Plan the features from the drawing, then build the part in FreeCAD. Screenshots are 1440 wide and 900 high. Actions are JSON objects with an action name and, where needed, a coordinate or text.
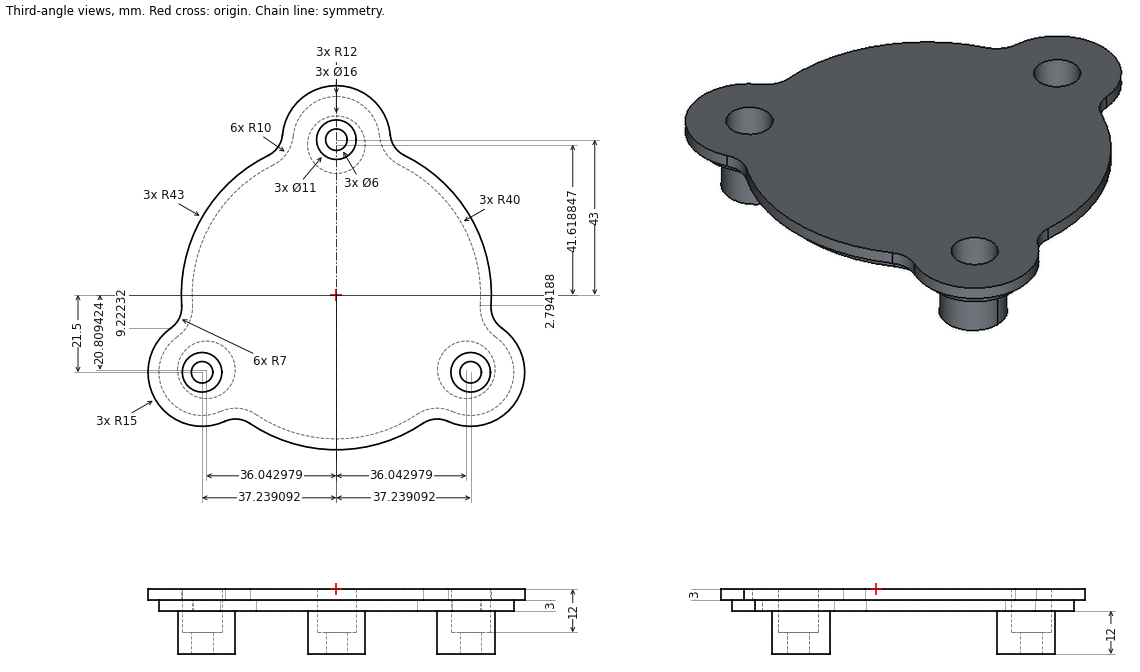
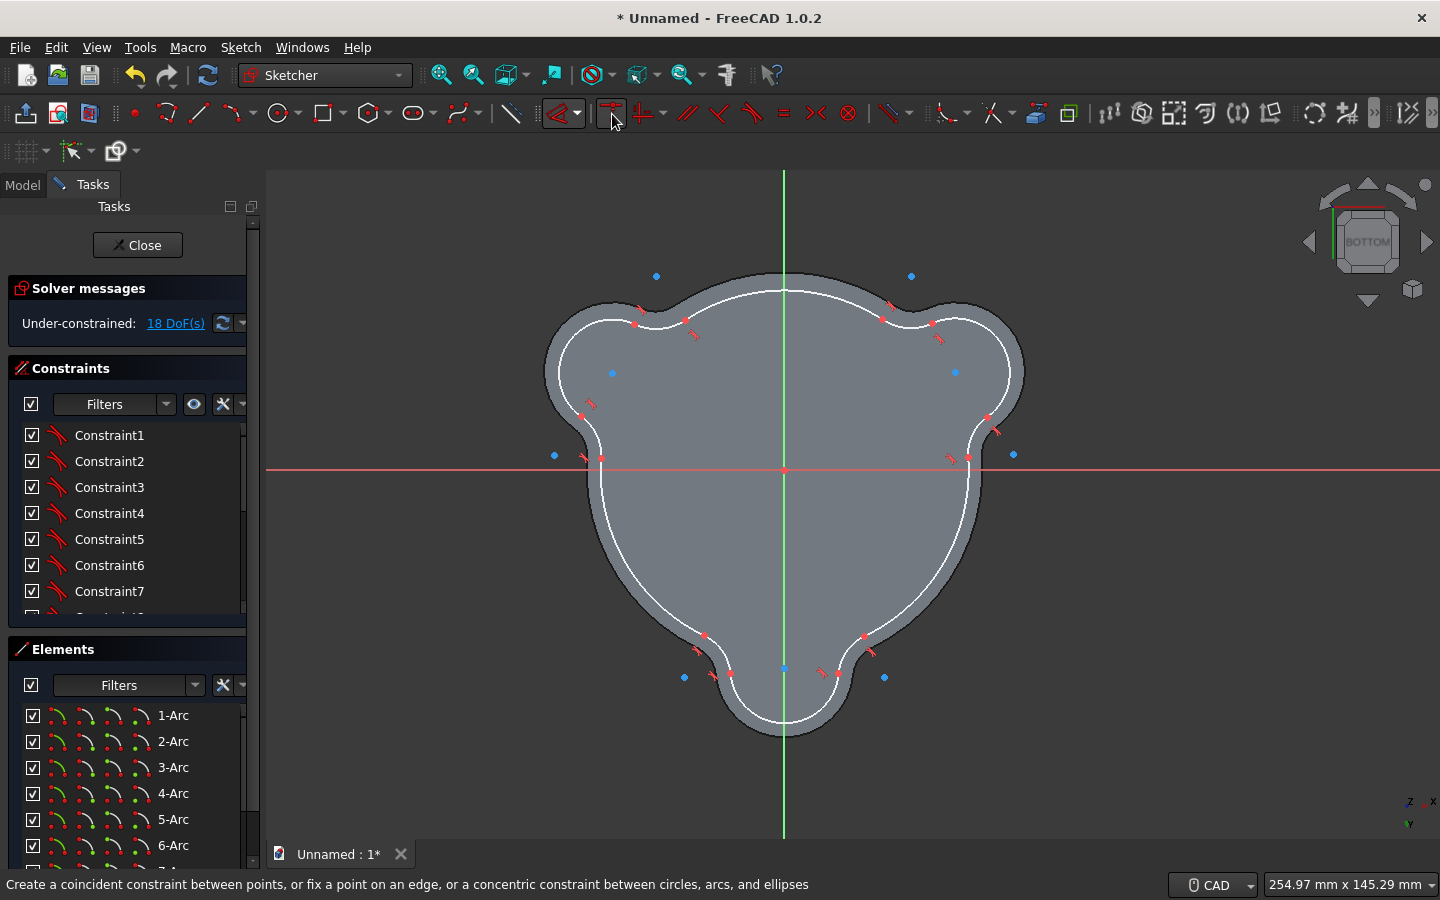
{"action": "left_click", "coordinate": [727, 660]}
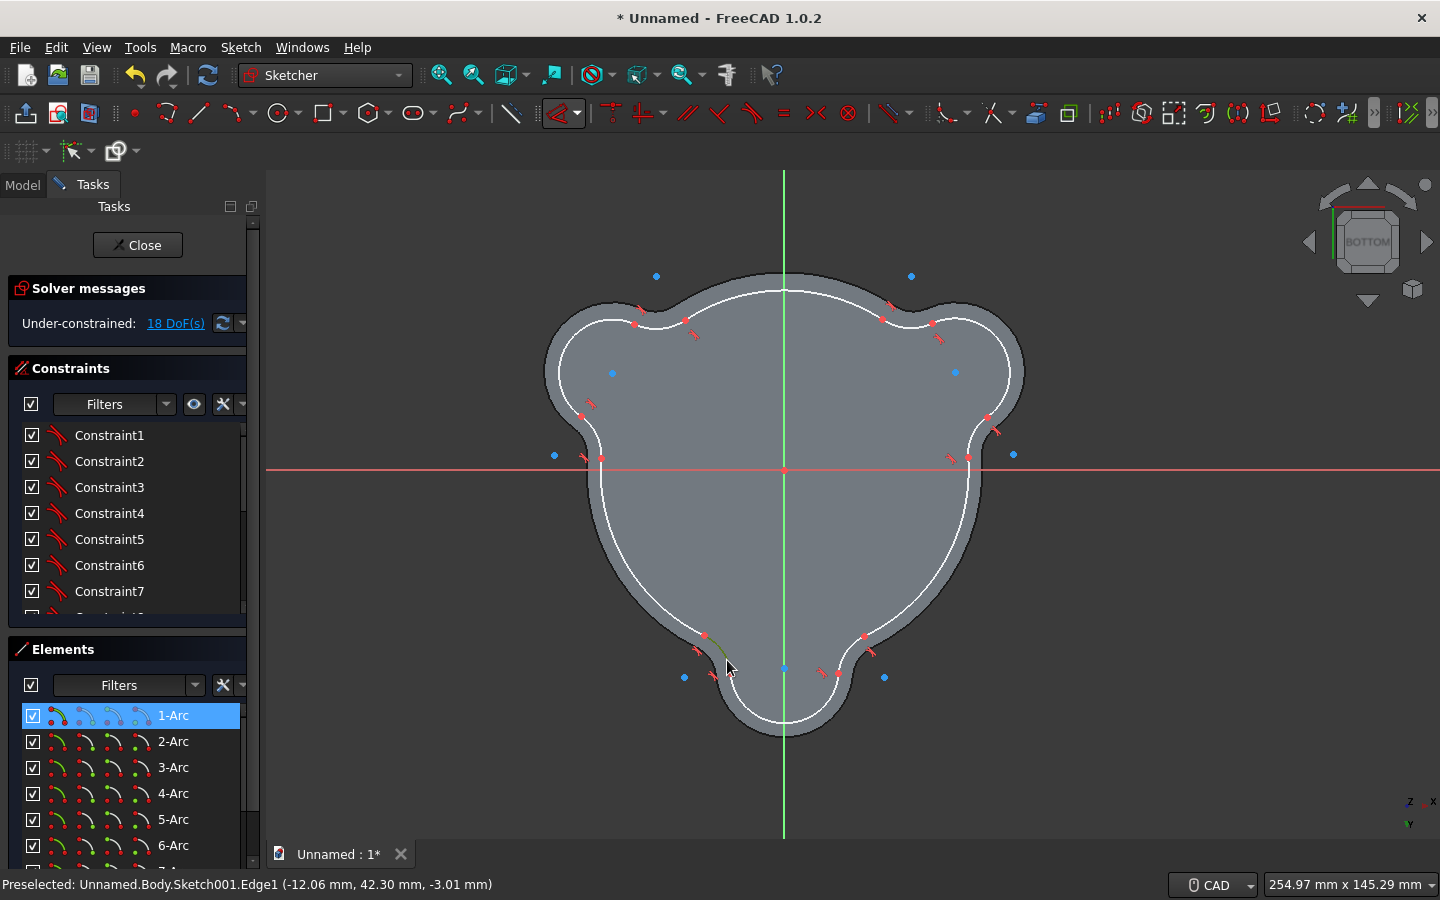
{"action": "left_click", "coordinate": [853, 644]}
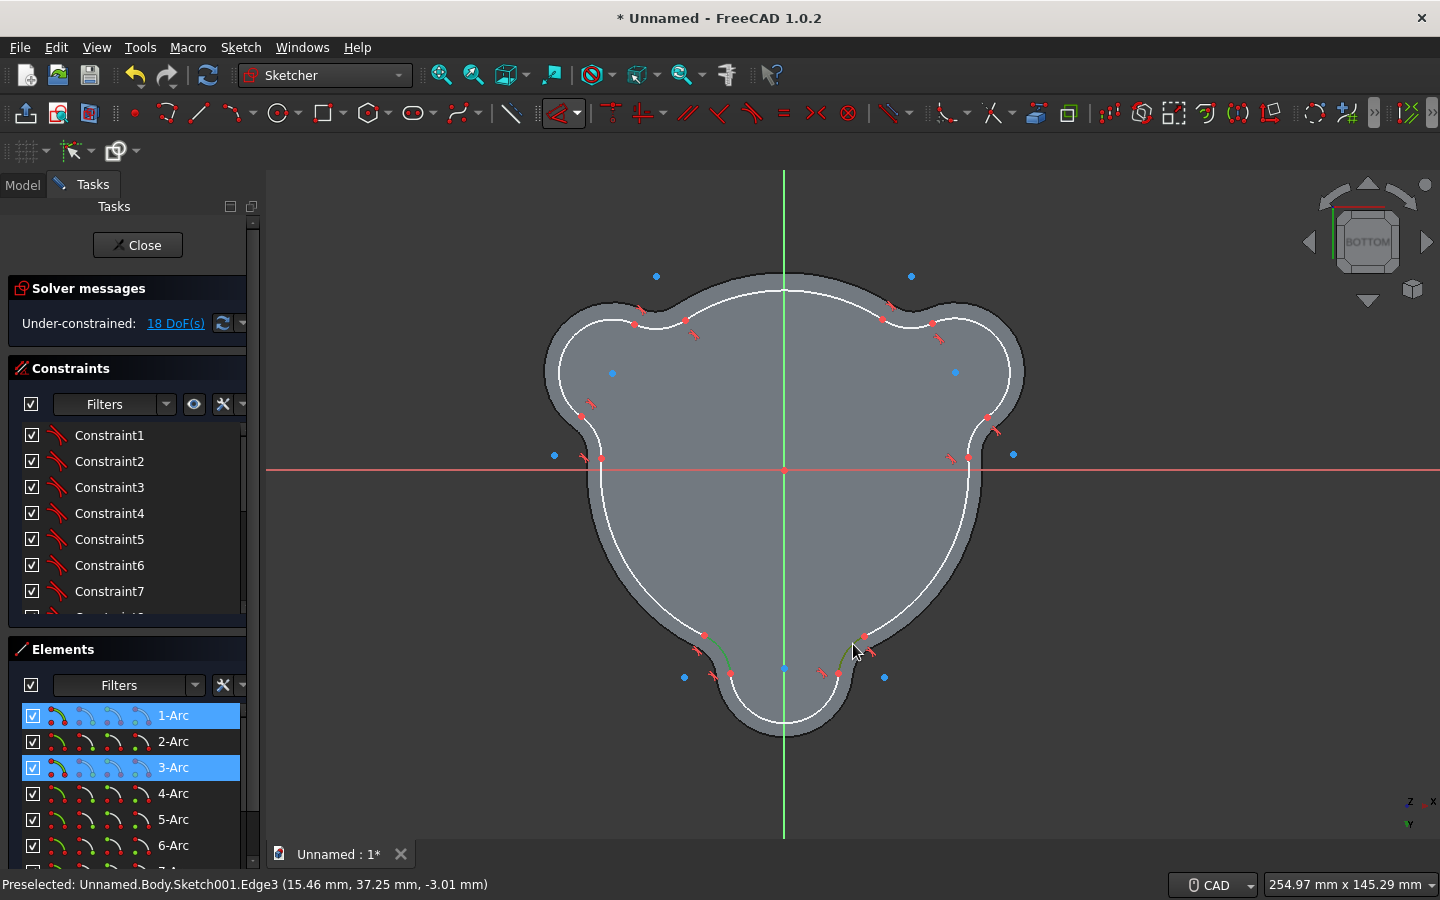
{"action": "left_click", "coordinate": [977, 427]}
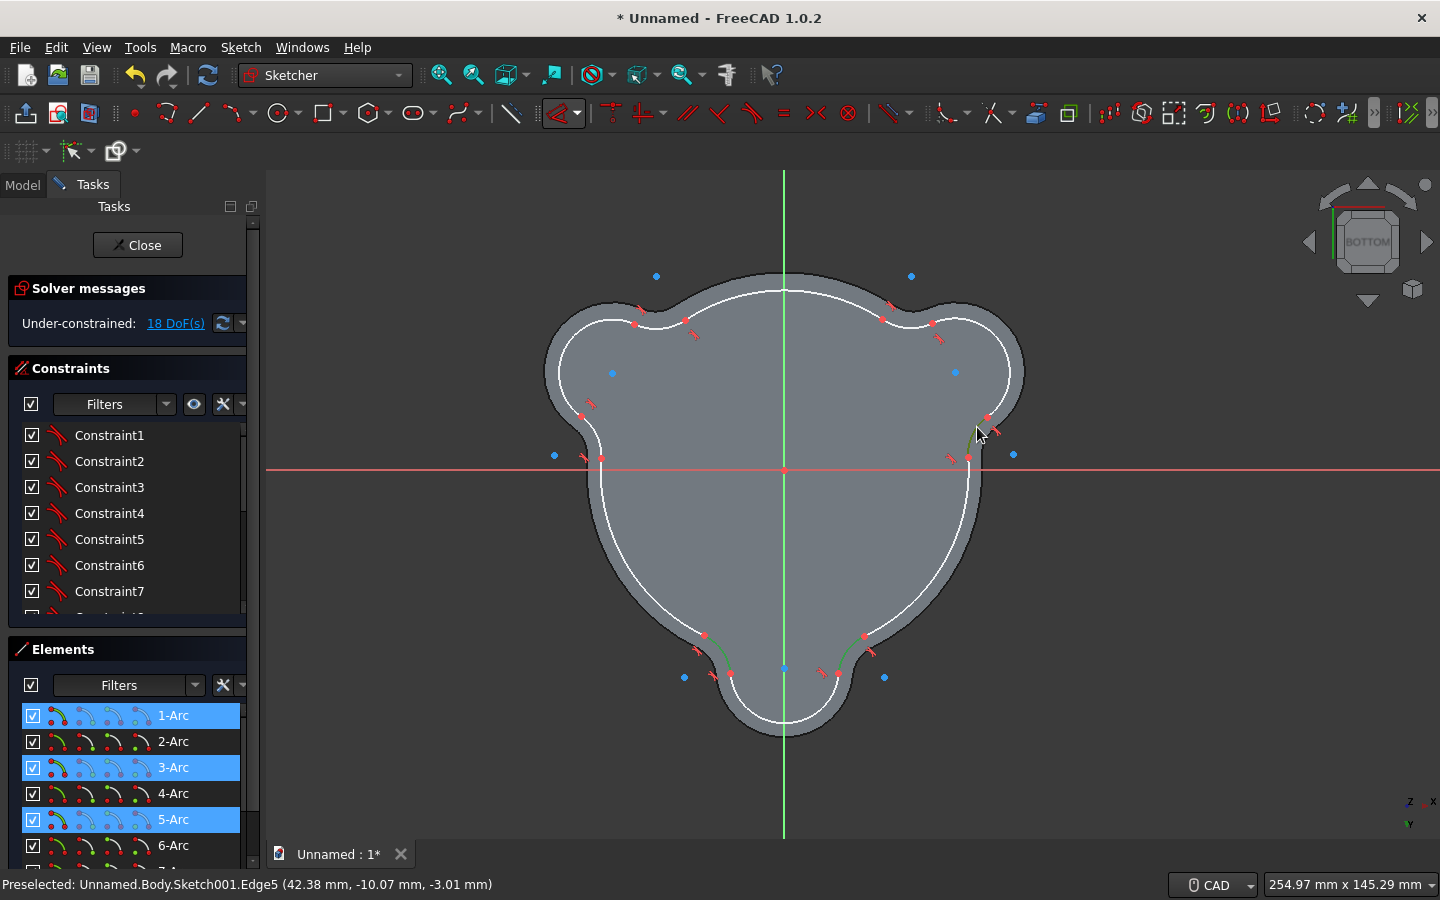
{"action": "left_click", "coordinate": [897, 326]}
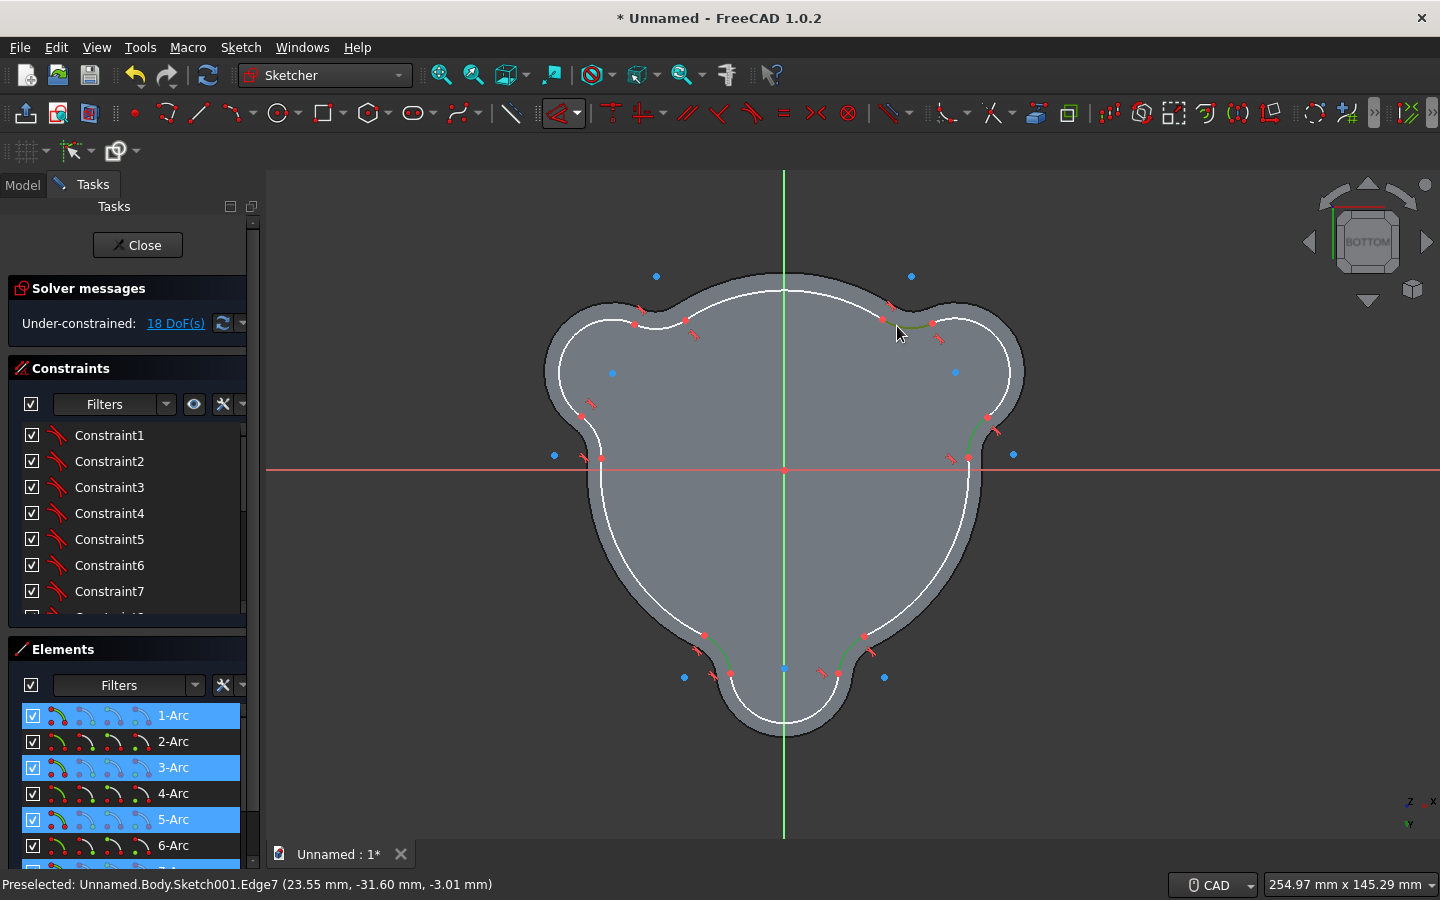
{"action": "left_click", "coordinate": [650, 329]}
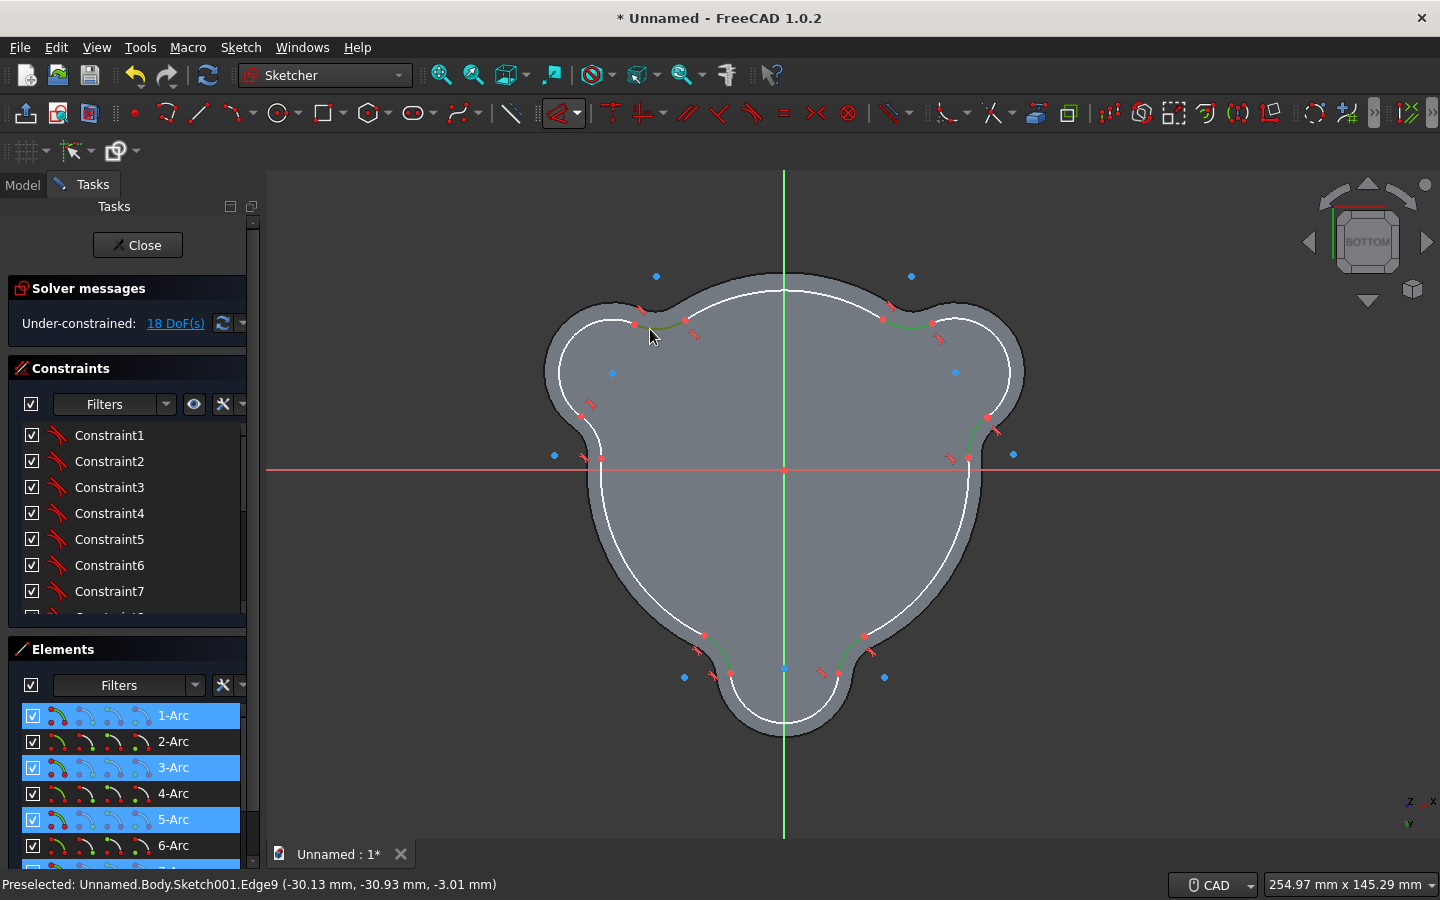
{"action": "left_click", "coordinate": [600, 444]}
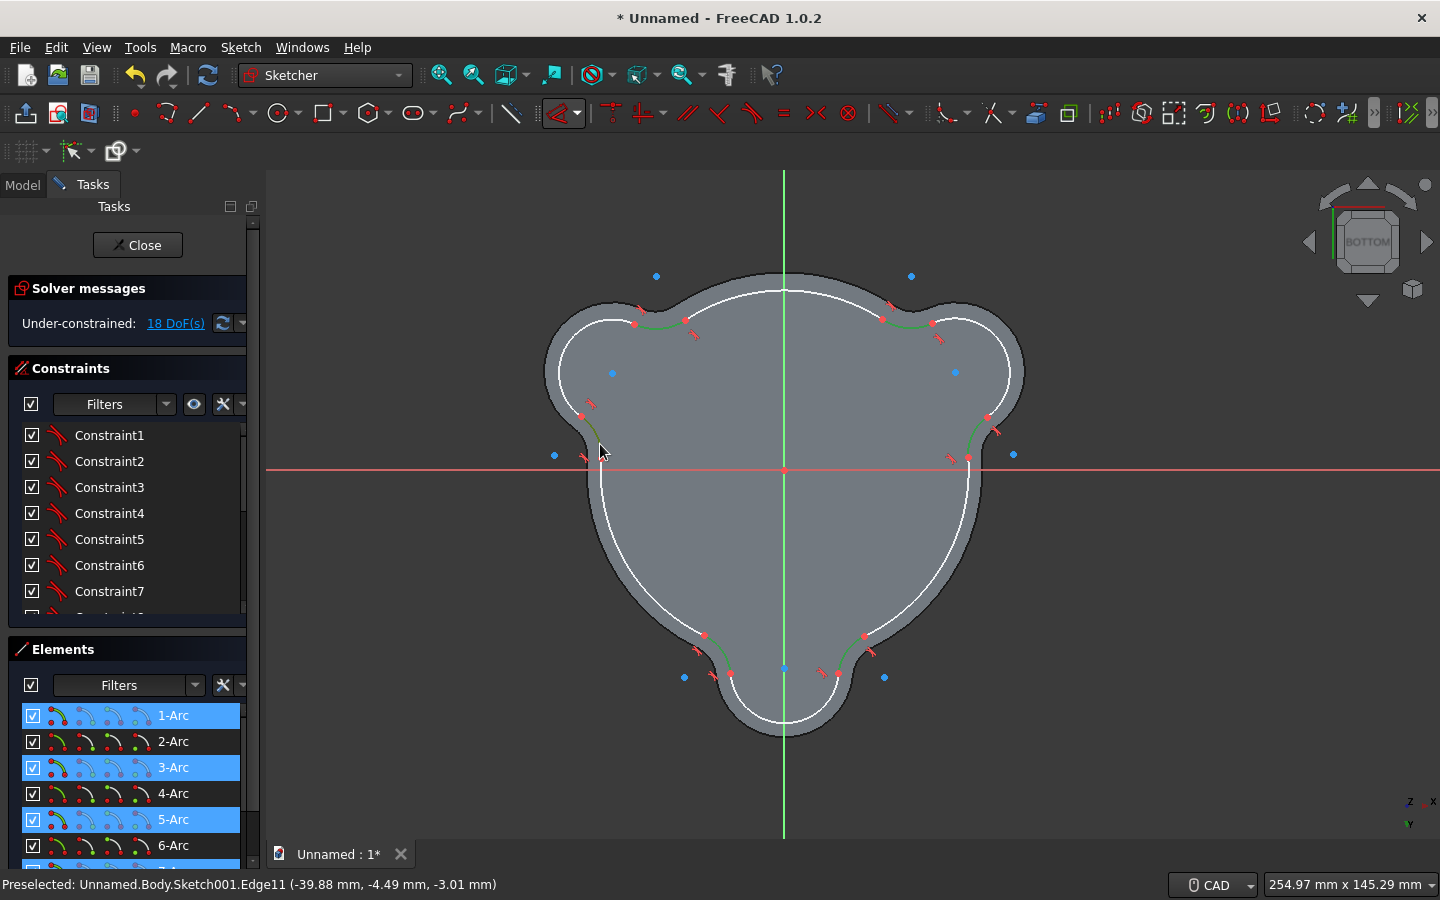
{"action": "left_click", "coordinate": [784, 114]}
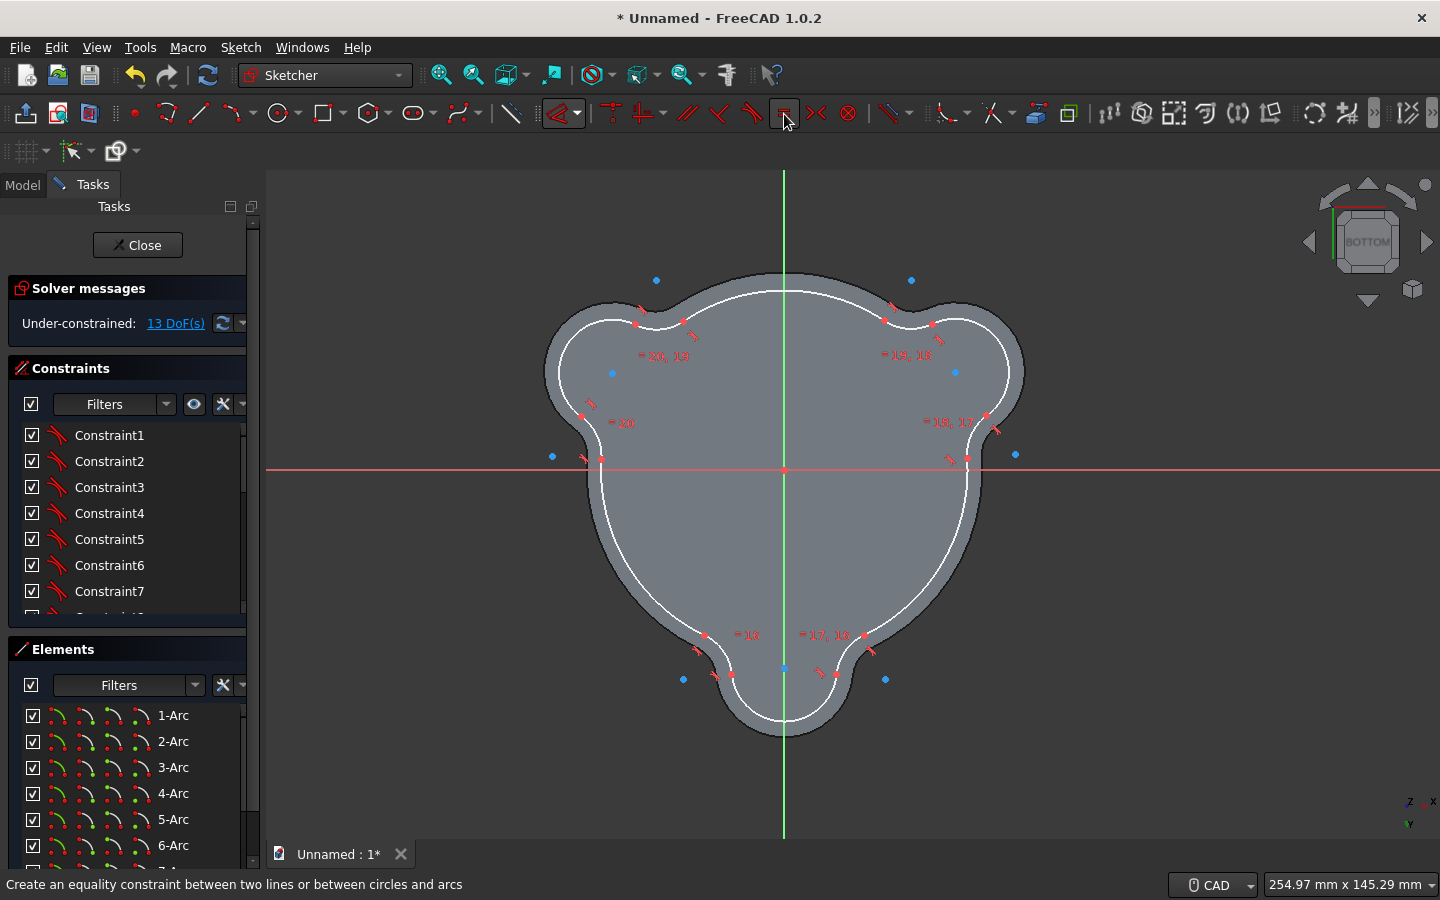
{"action": "left_click", "coordinate": [755, 713]}